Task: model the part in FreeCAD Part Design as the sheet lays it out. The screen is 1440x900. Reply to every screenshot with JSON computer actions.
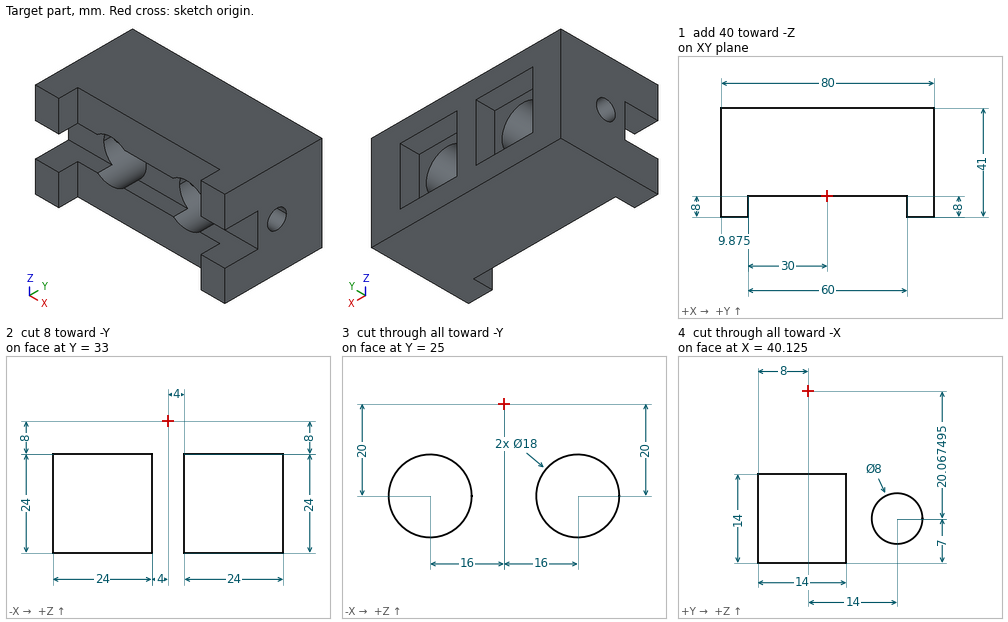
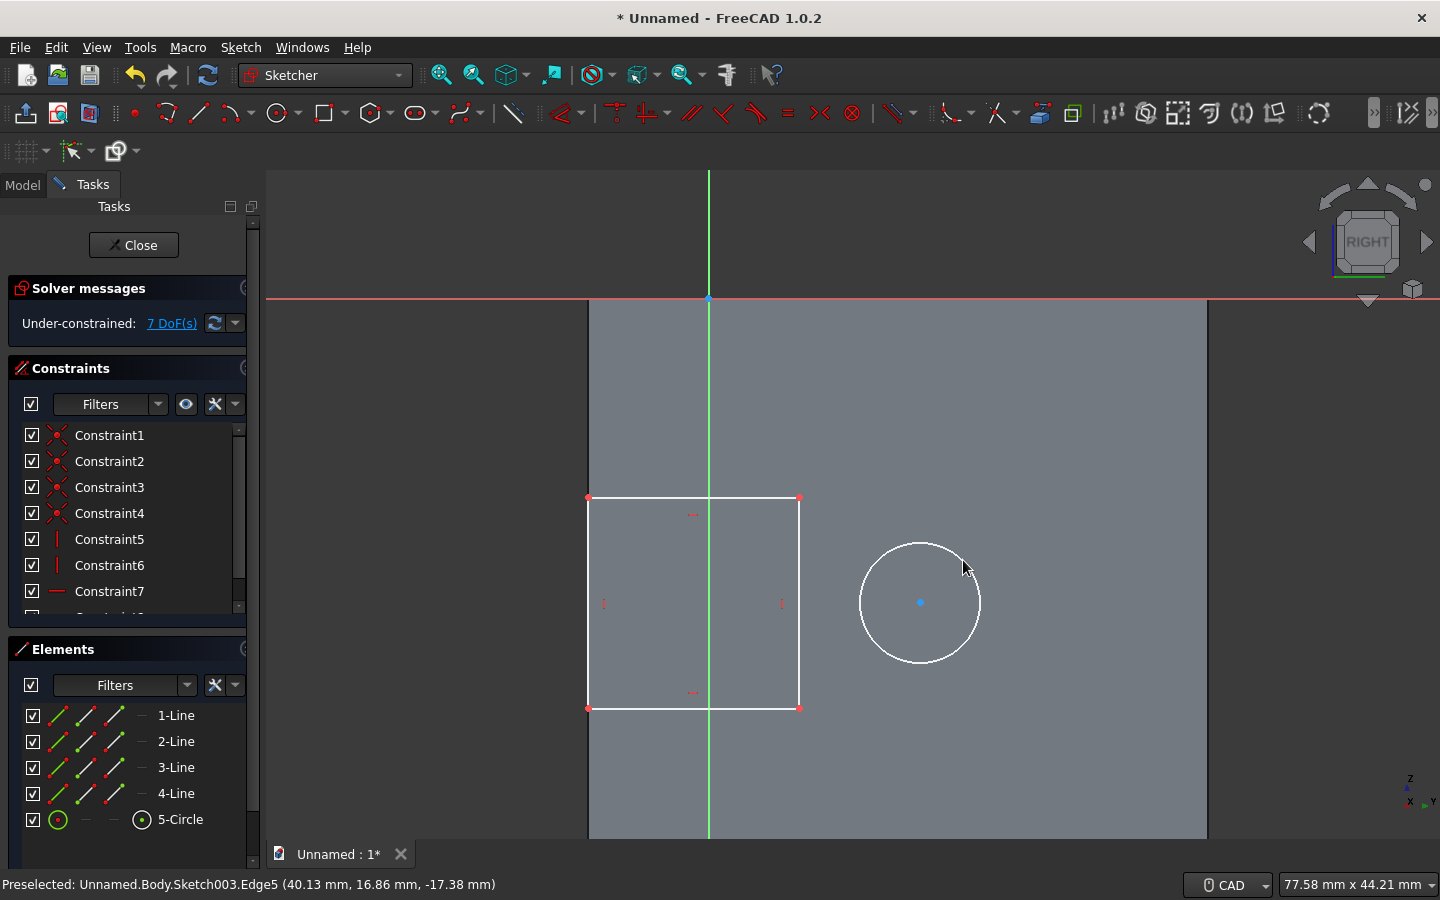
{"action": "key", "text": "d"}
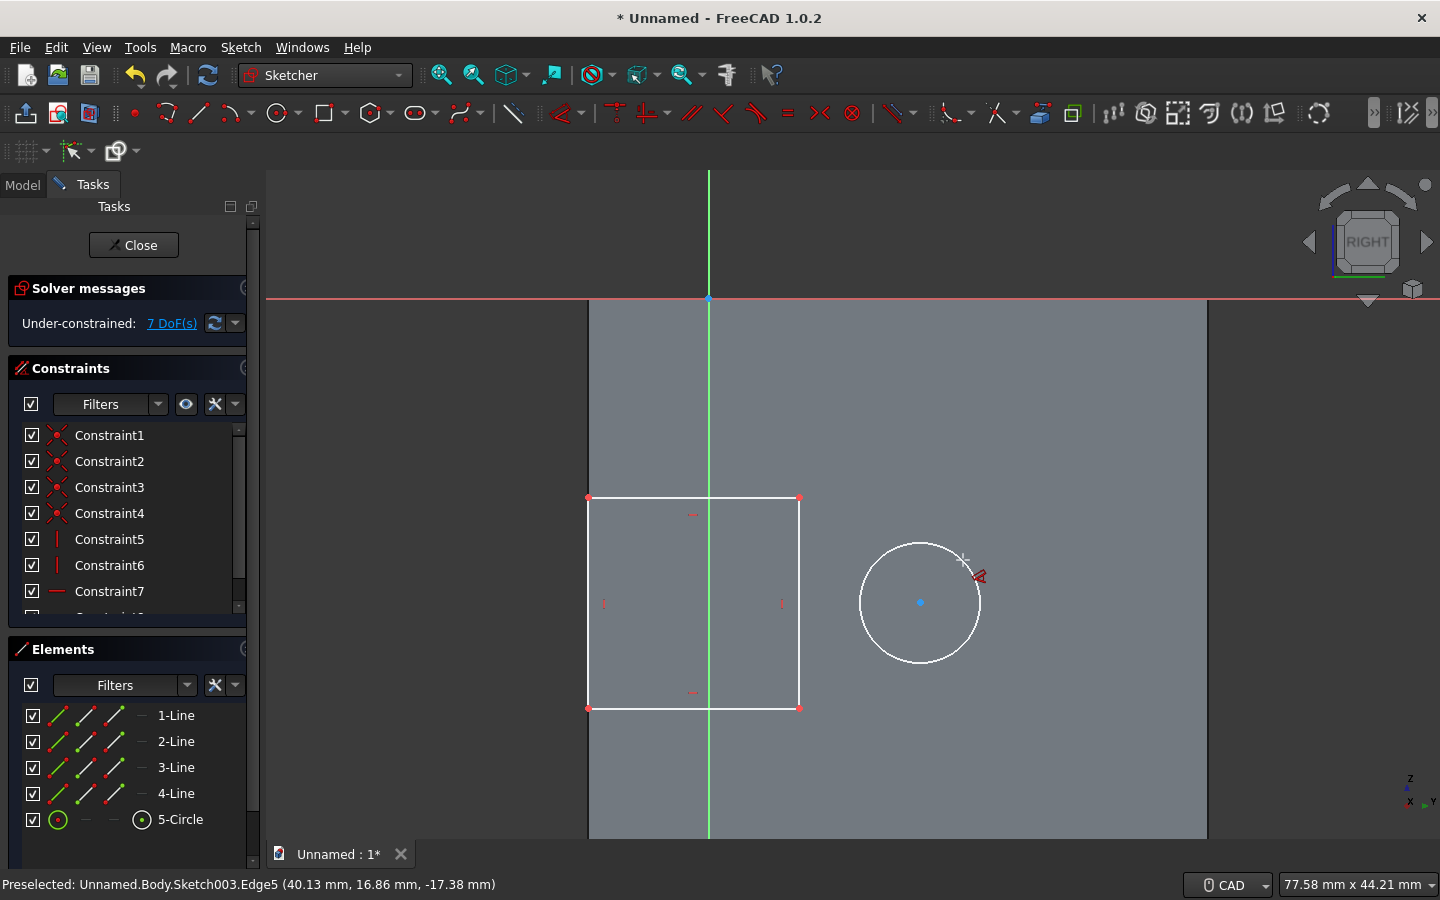
{"action": "left_click", "coordinate": [962, 560]}
{"action": "left_click", "coordinate": [984, 537]}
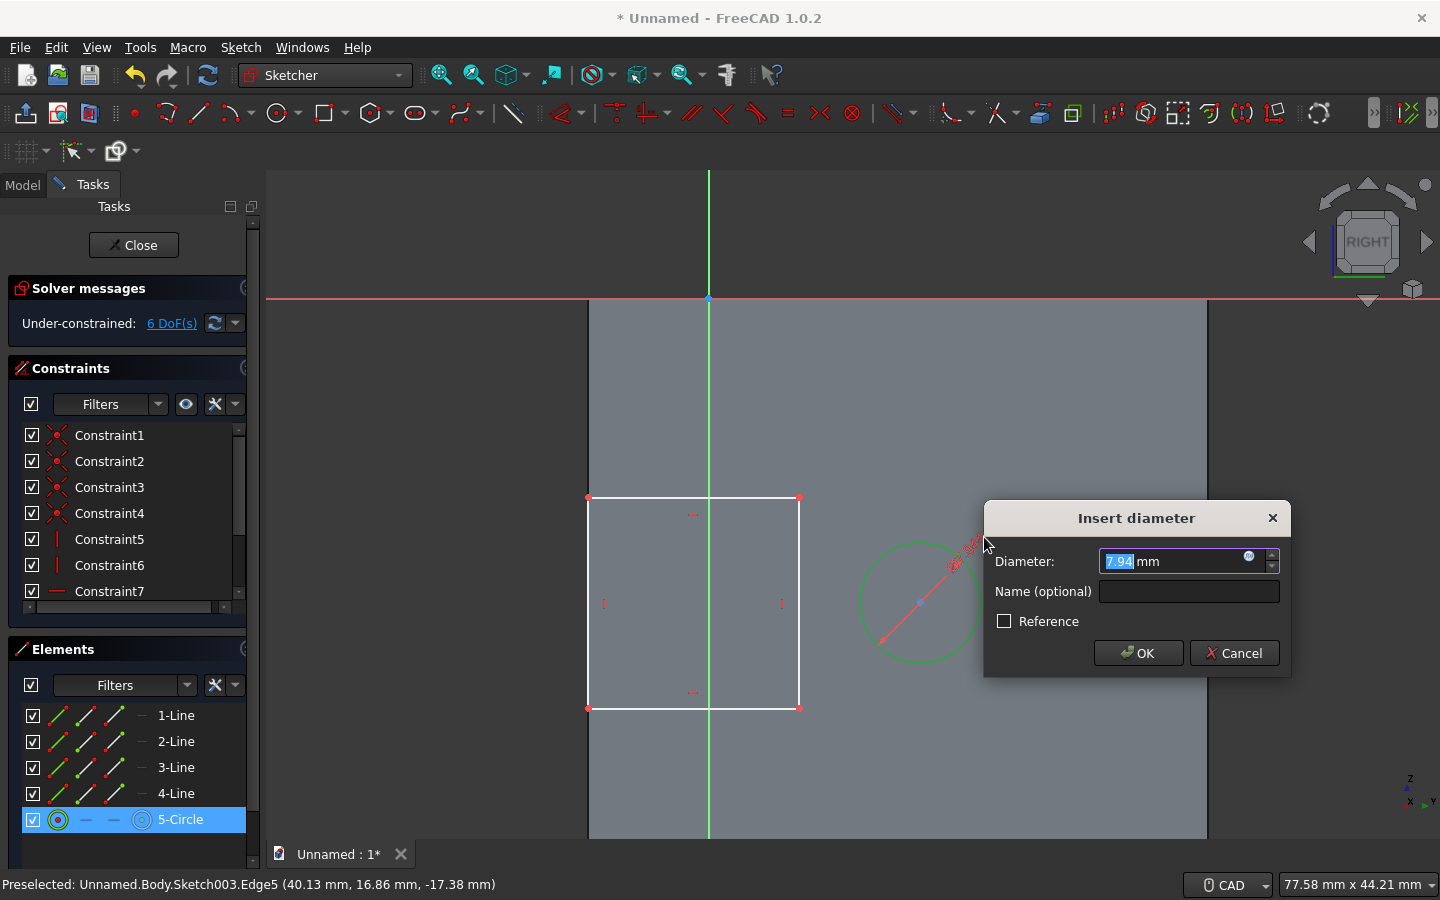
{"action": "type", "text": "8"}
{"action": "key", "text": "Return"}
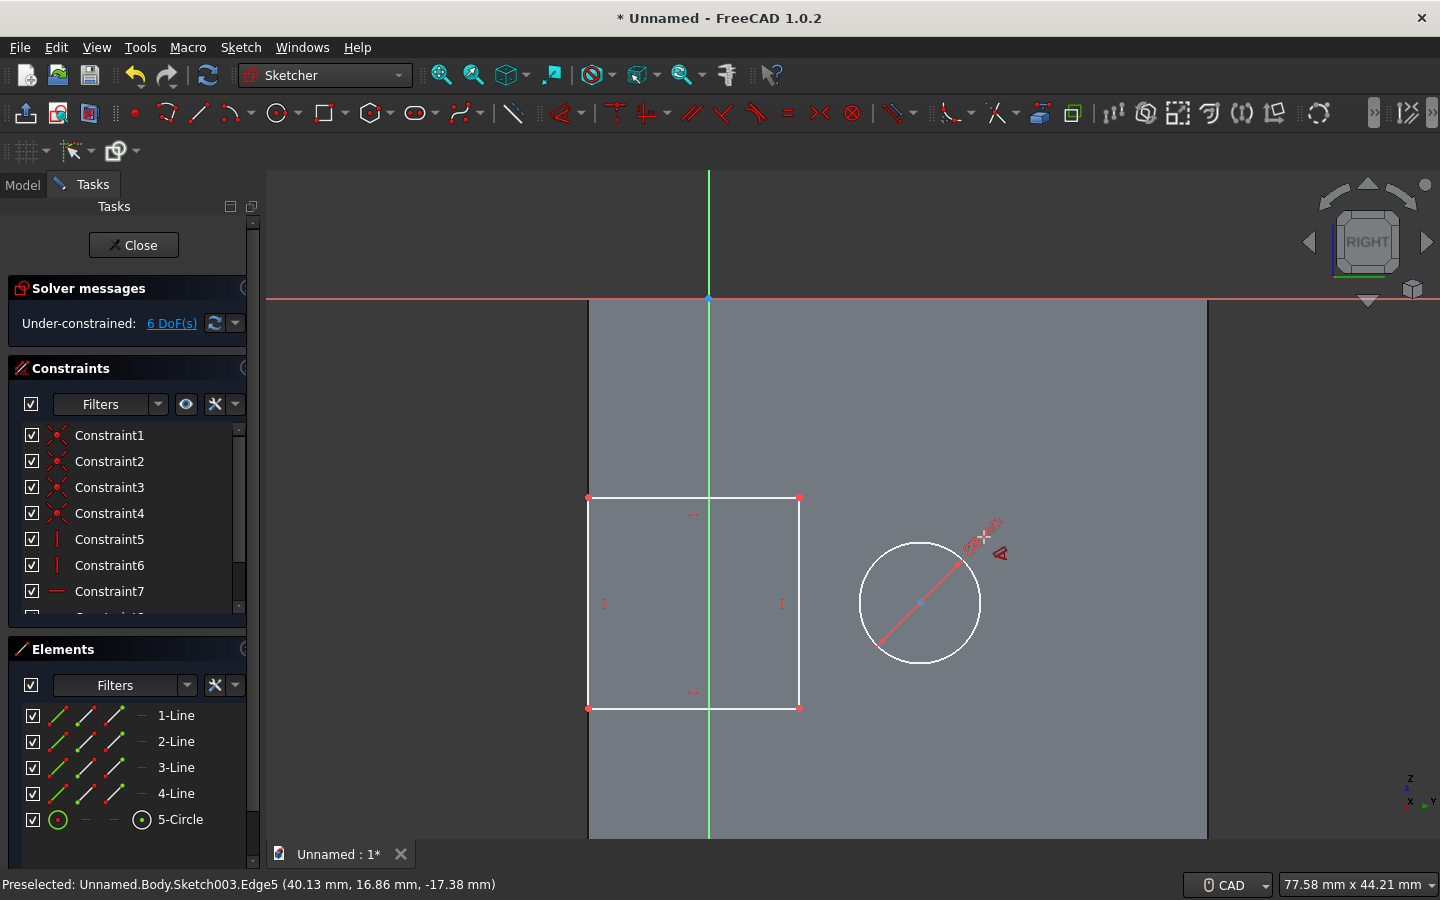
{"action": "left_click", "coordinate": [588, 561]}
{"action": "left_click", "coordinate": [554, 604]}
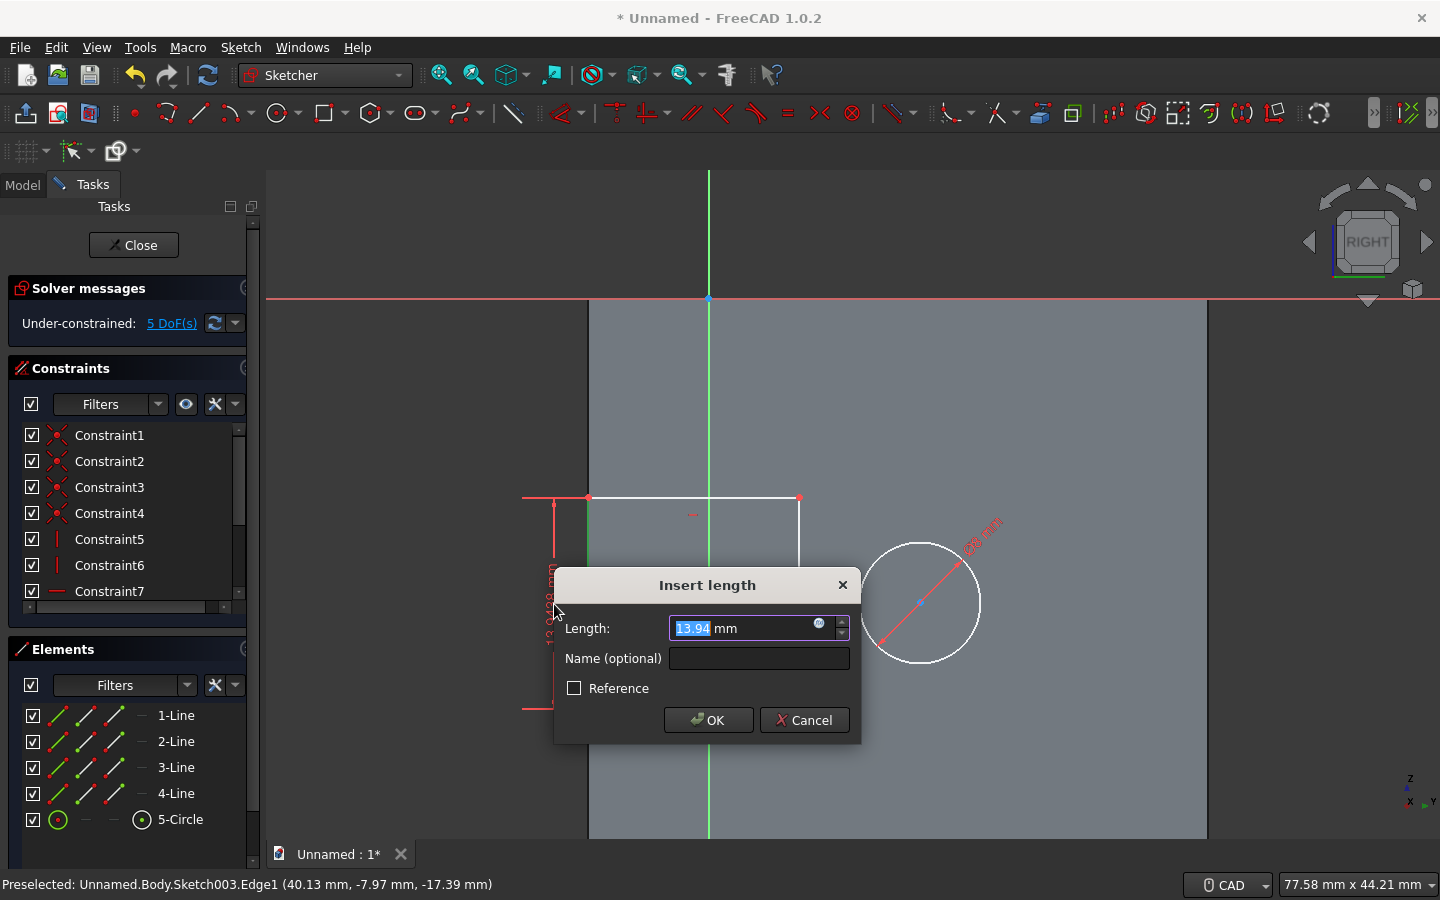
{"action": "type", "text": "14"}
{"action": "key", "text": "Return"}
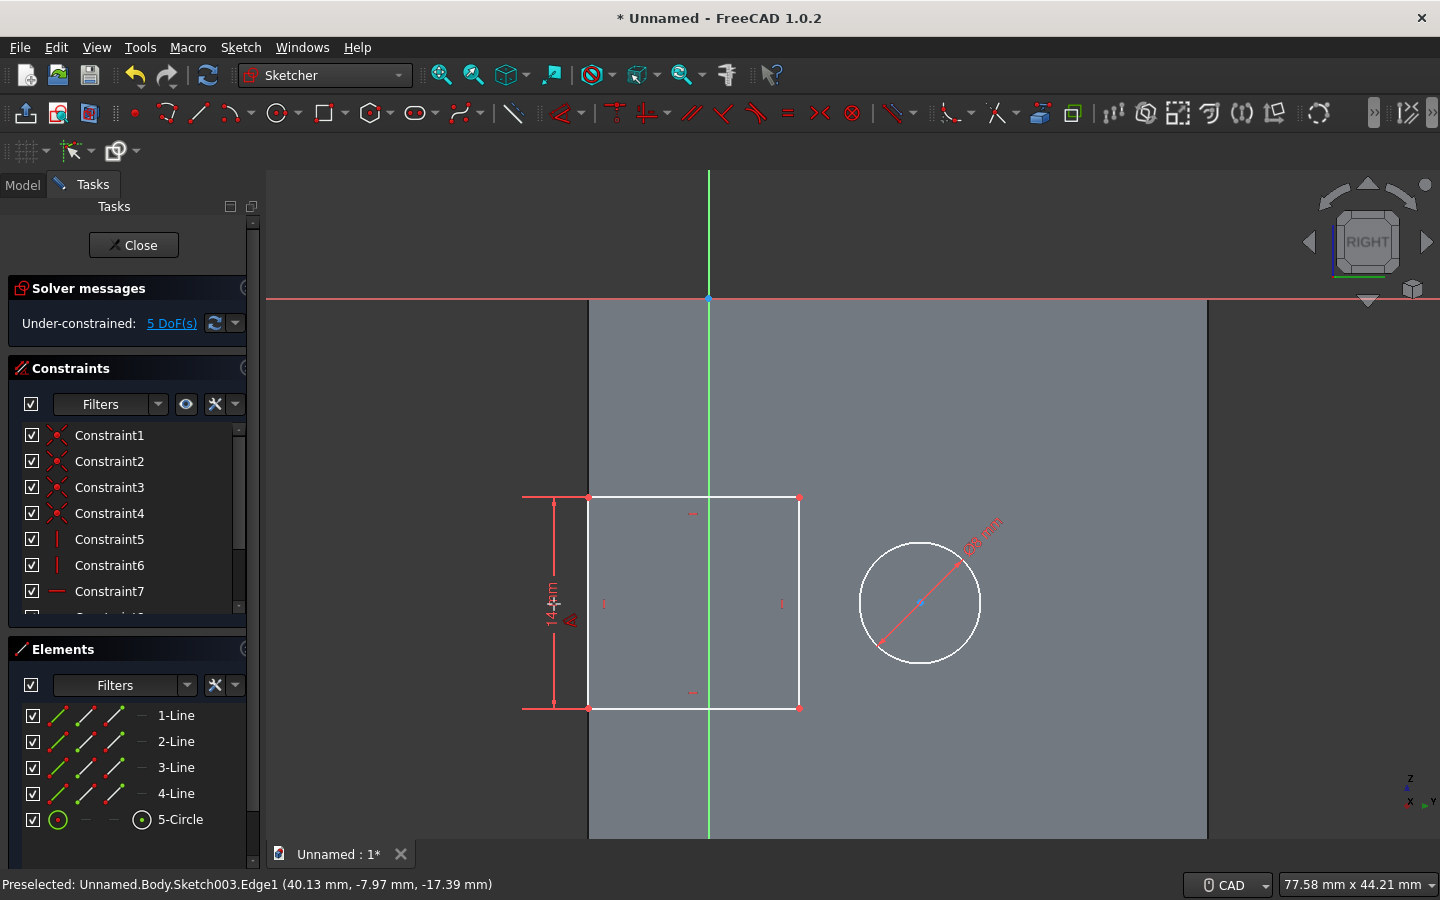
{"action": "left_click", "coordinate": [651, 709]}
{"action": "left_click", "coordinate": [693, 743]}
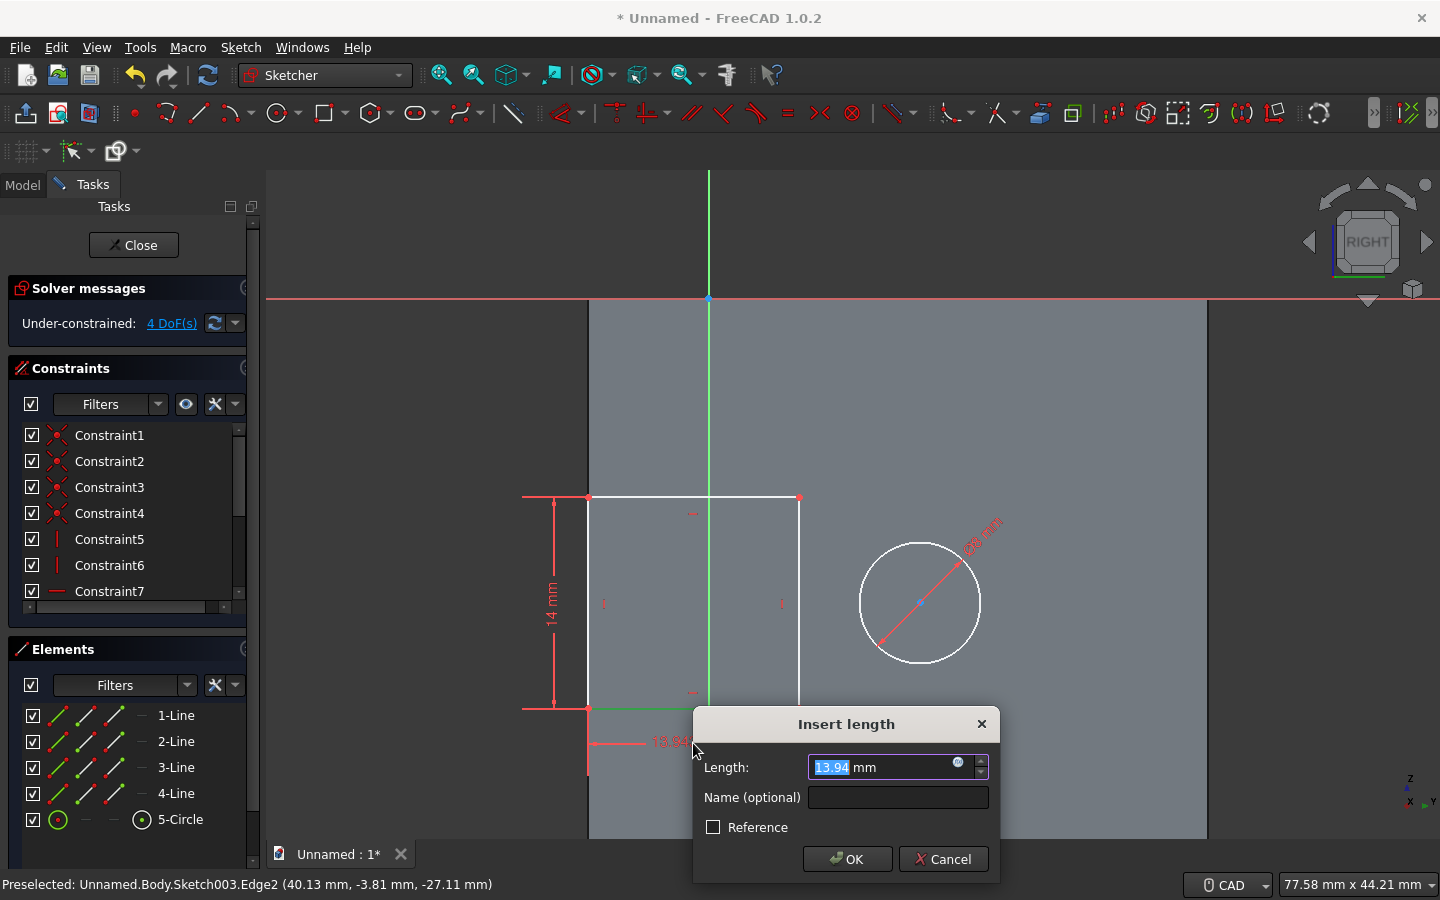
{"action": "type", "text": "14"}
{"action": "key", "text": "Return"}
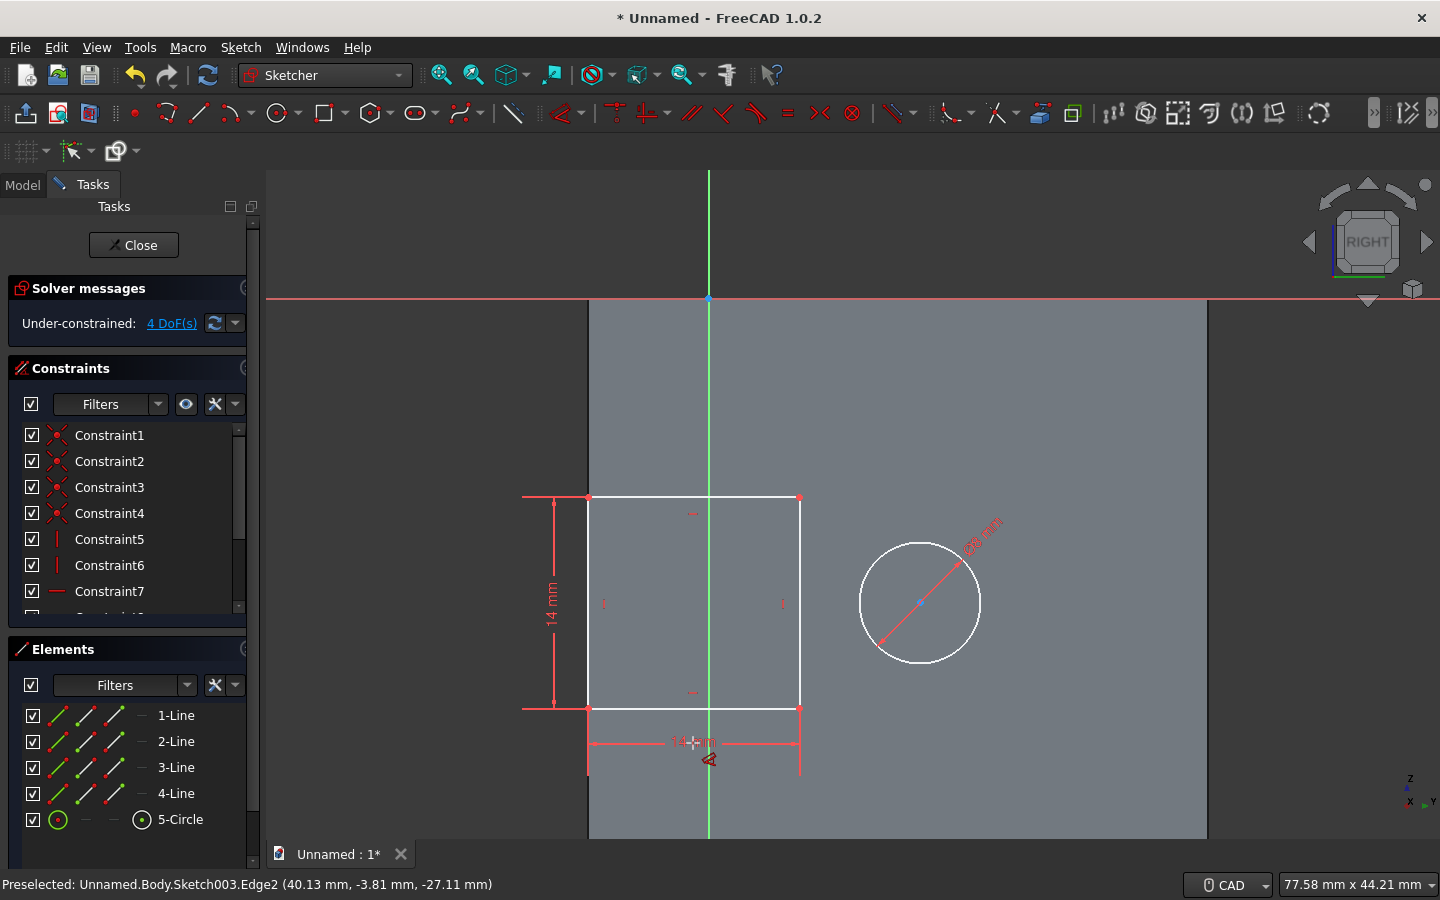
{"action": "left_click", "coordinate": [588, 497]}
{"action": "left_click", "coordinate": [648, 265]}